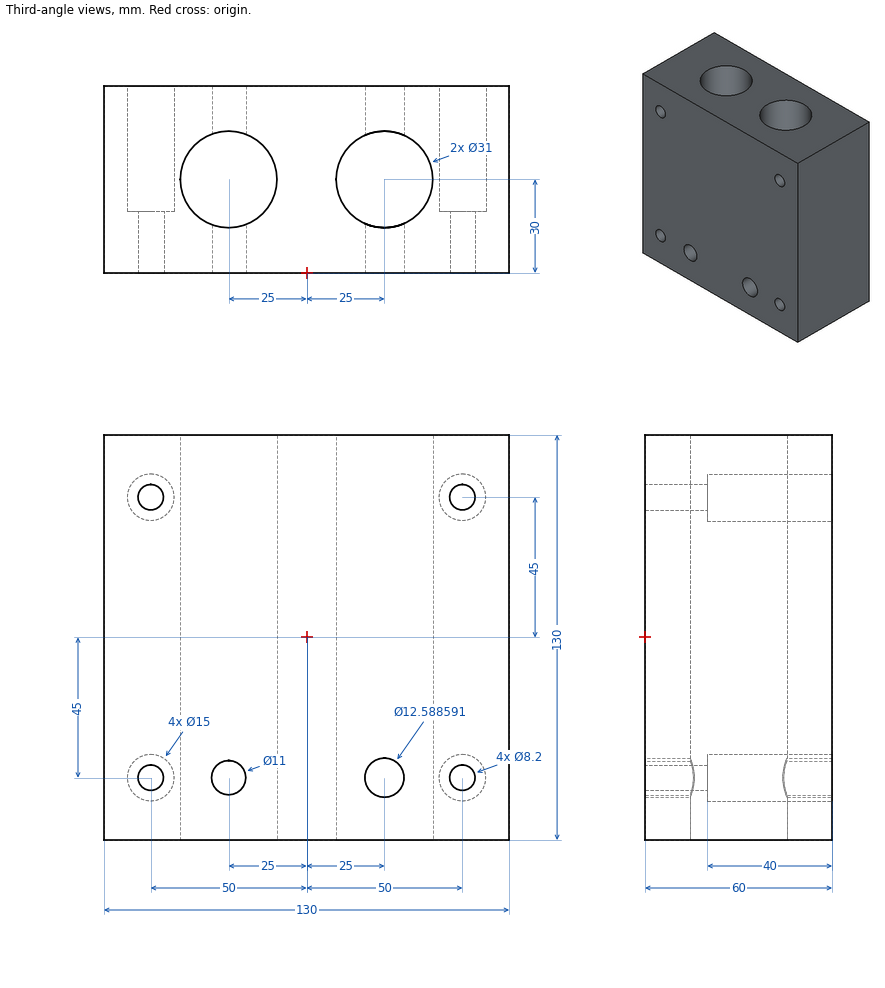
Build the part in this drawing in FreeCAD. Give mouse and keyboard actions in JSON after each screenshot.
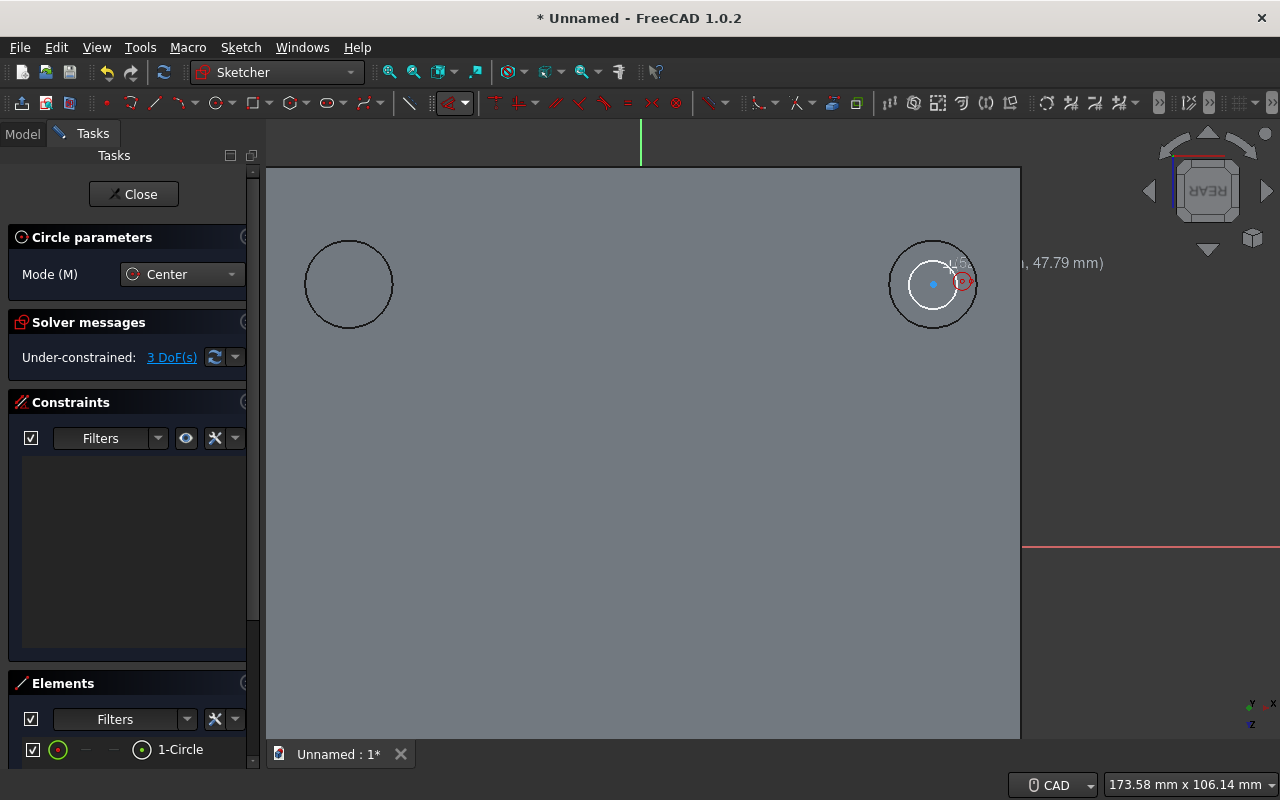
{"action": "left_click", "coordinate": [349, 284]}
{"action": "left_click", "coordinate": [366, 267]}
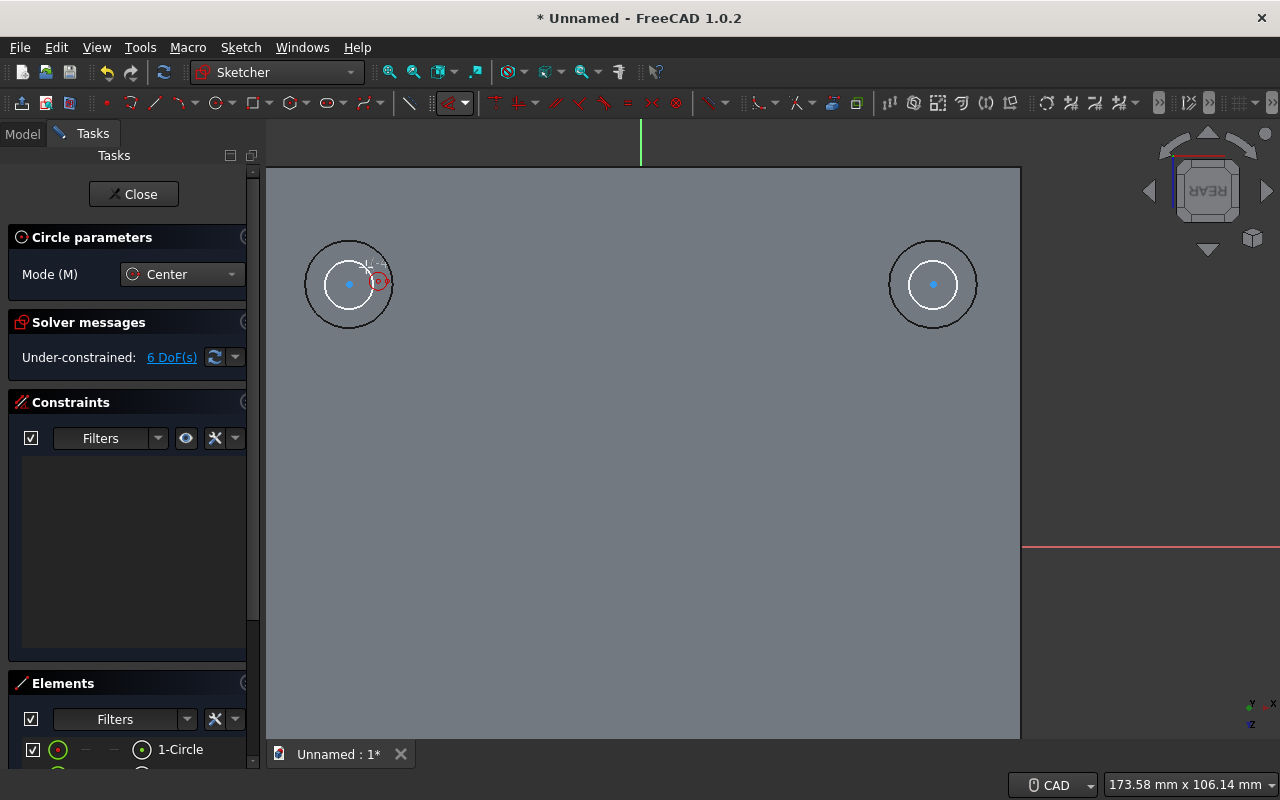
{"action": "scroll", "coordinate": [834, 189], "scroll_direction": "down", "scroll_amount": 2}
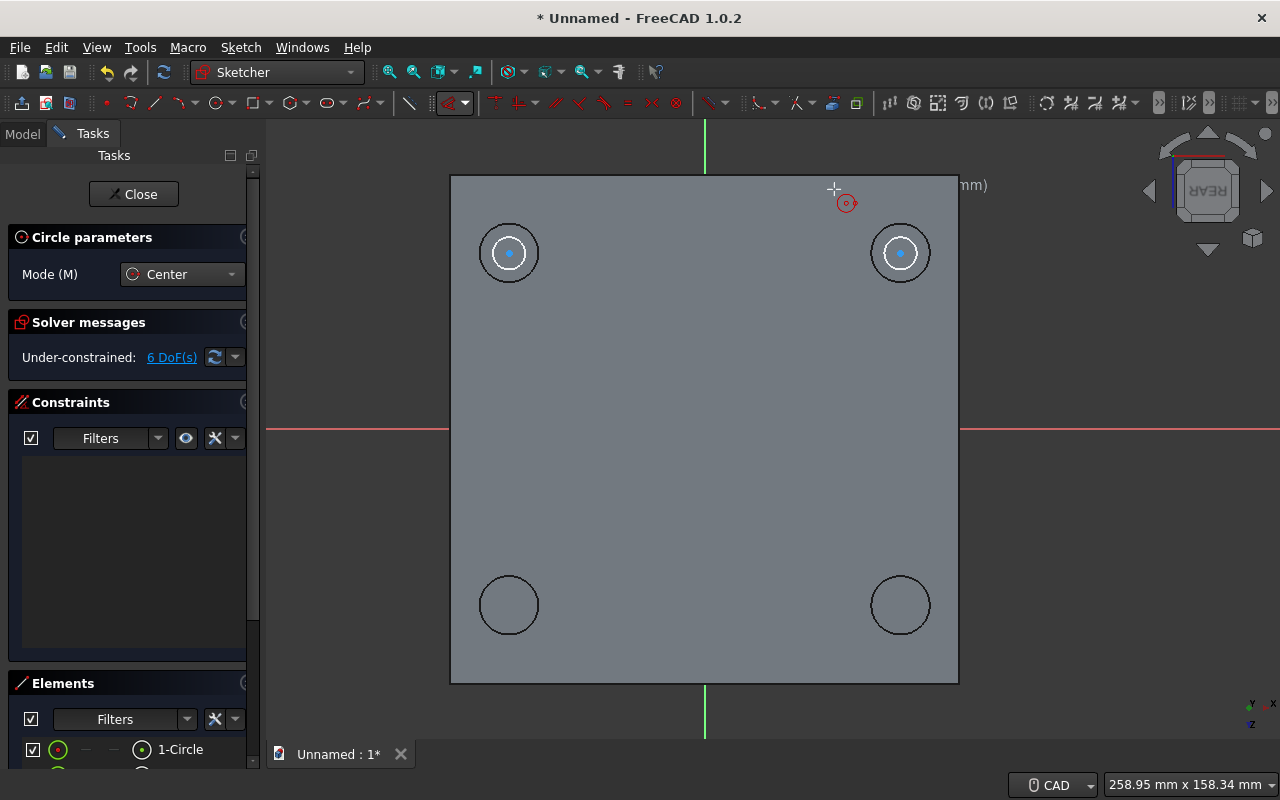
{"action": "scroll", "coordinate": [509, 605], "scroll_direction": "up", "scroll_amount": 2}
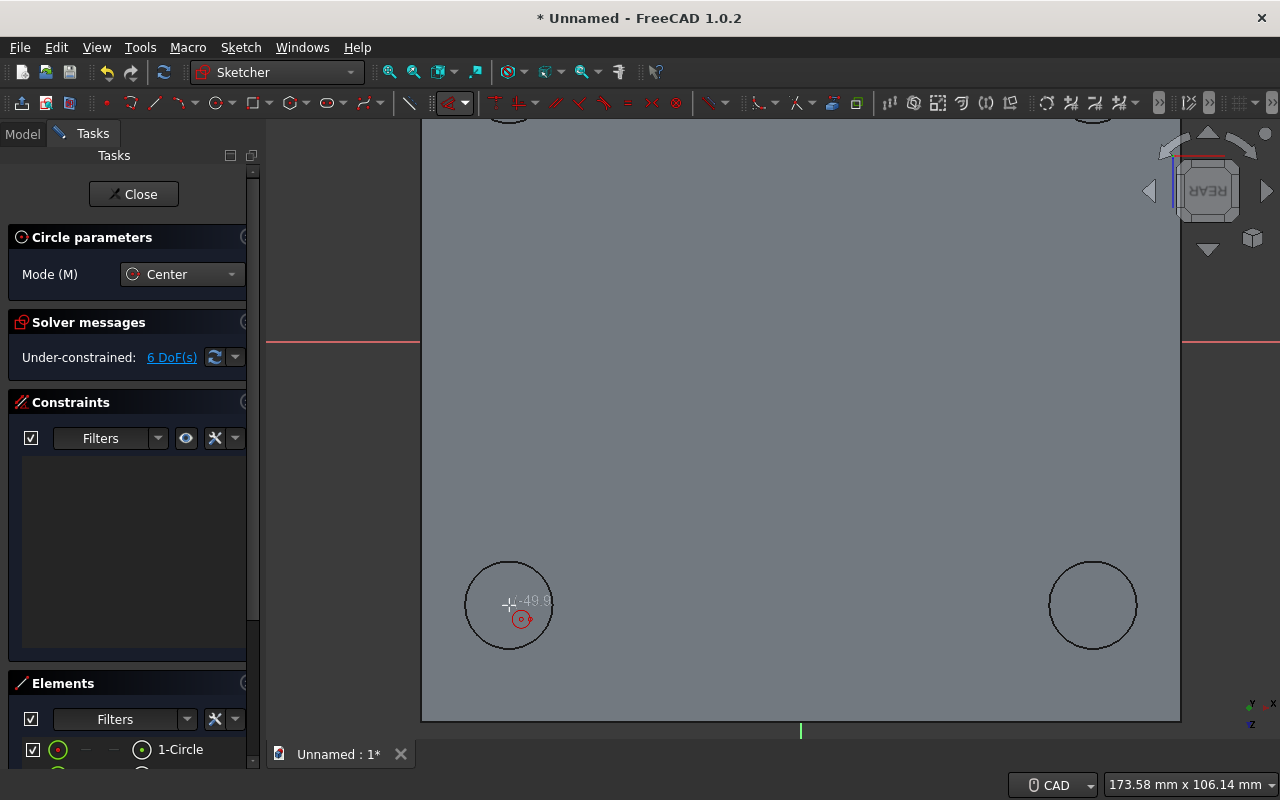
{"action": "left_click", "coordinate": [509, 605]}
{"action": "left_click", "coordinate": [526, 588]}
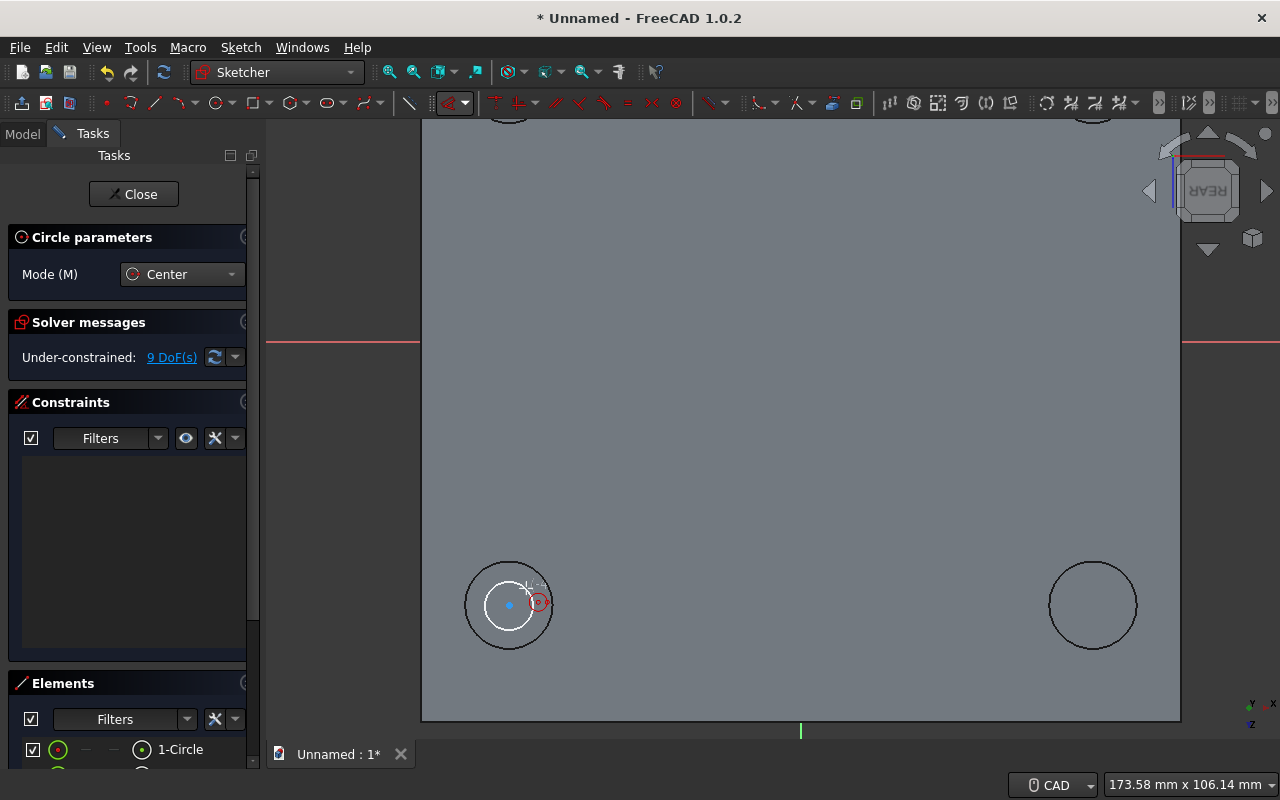
{"action": "left_click", "coordinate": [1093, 605]}
{"action": "left_click", "coordinate": [1110, 588]}
{"action": "key", "text": "Escape"}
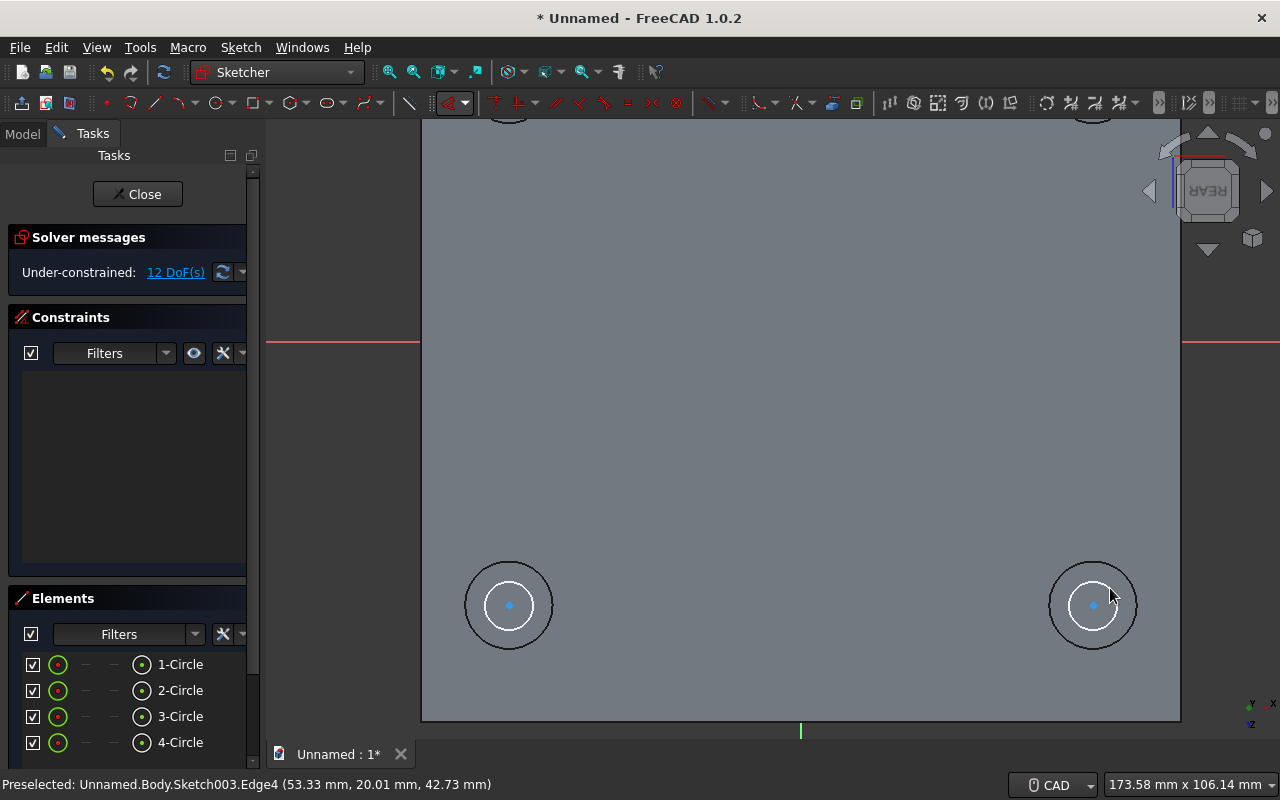
{"action": "scroll", "coordinate": [508, 605], "scroll_direction": "down", "scroll_amount": 2}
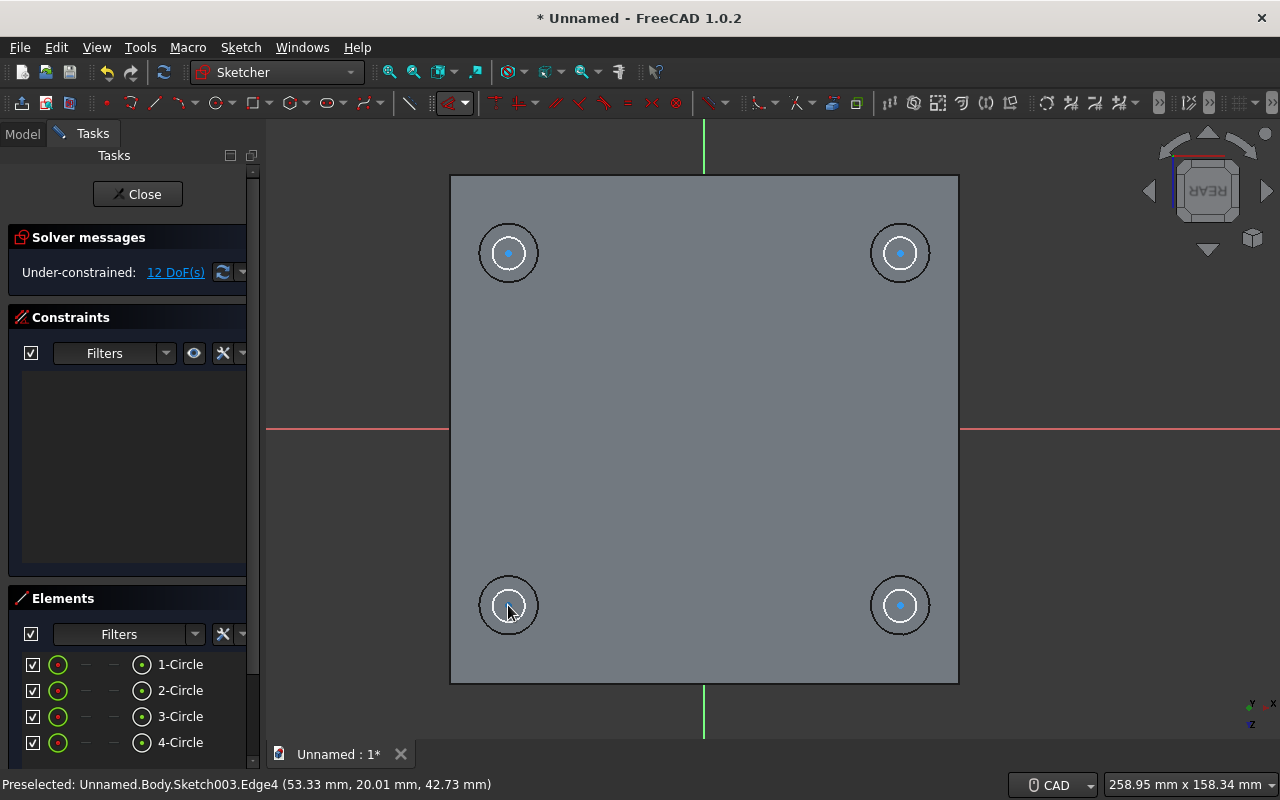
{"action": "left_click", "coordinate": [912, 242]}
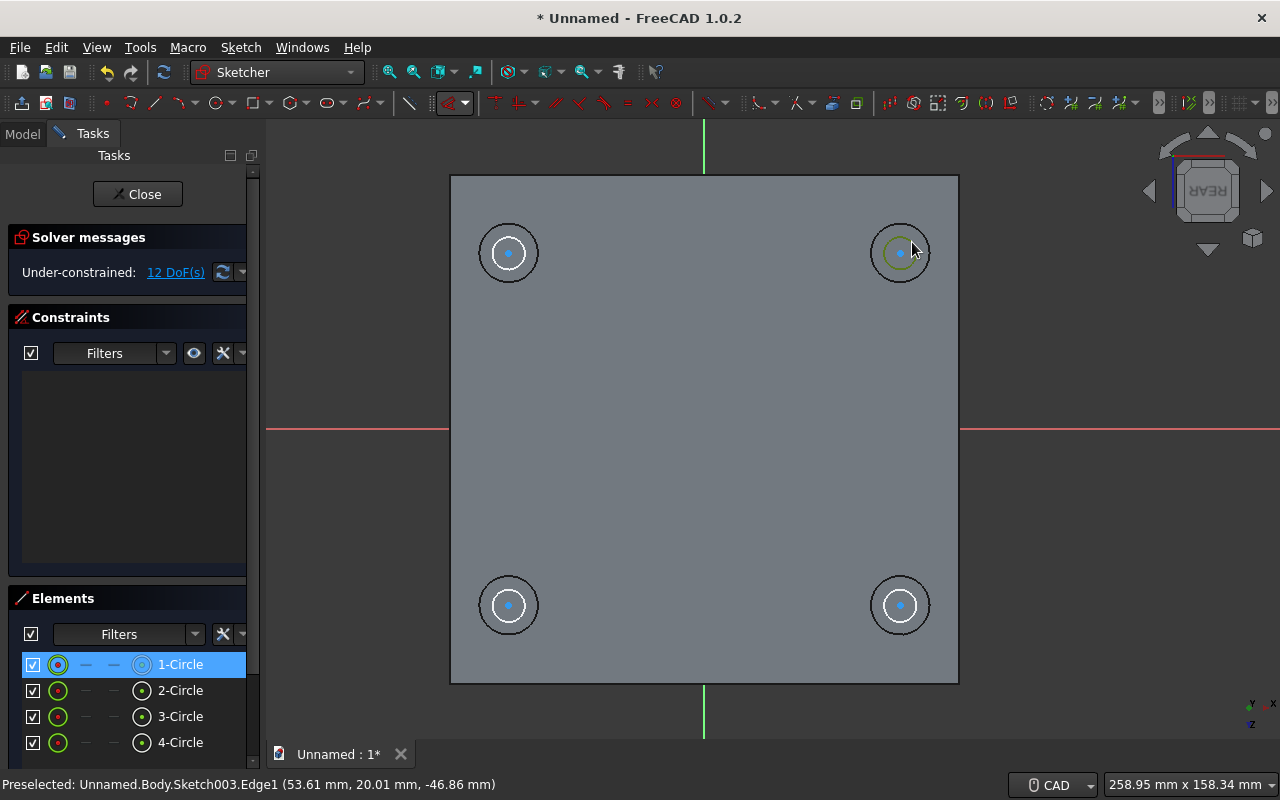
{"action": "left_click", "coordinate": [520, 242]}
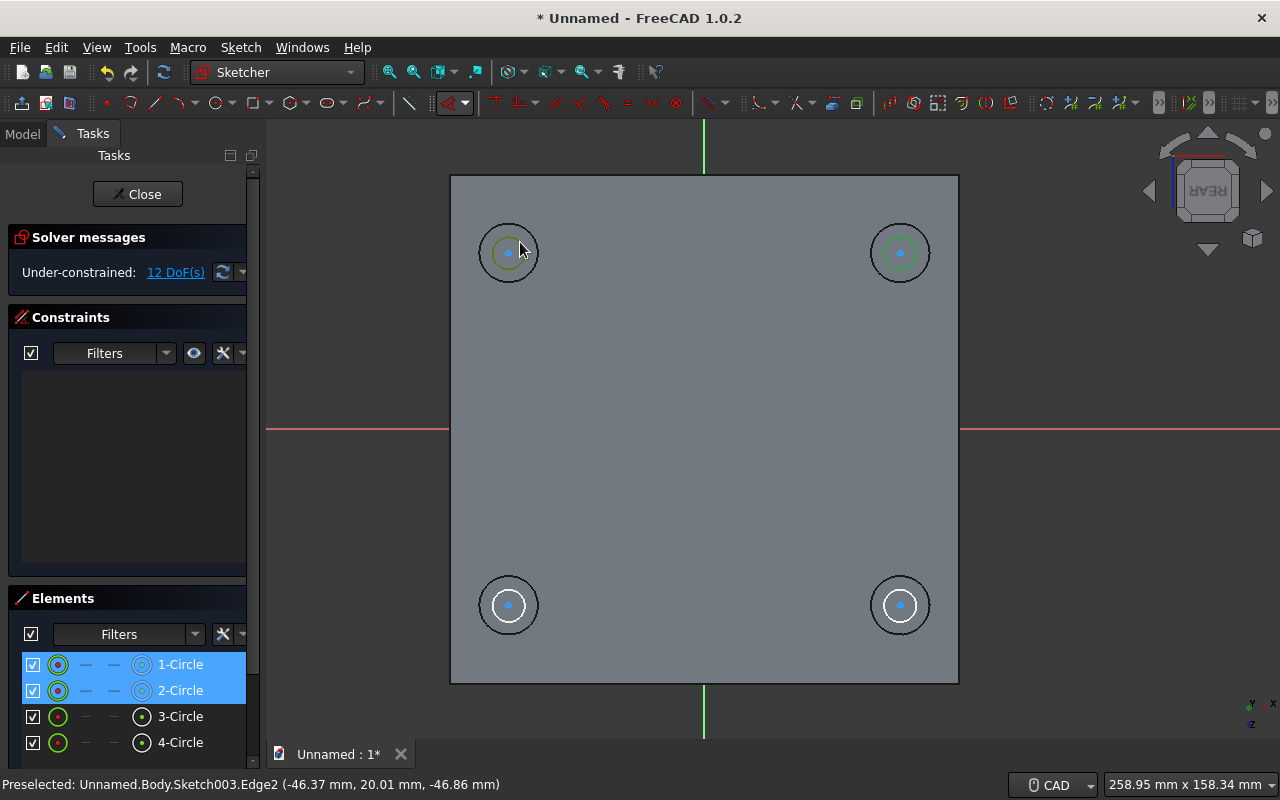
{"action": "left_click", "coordinate": [520, 594]}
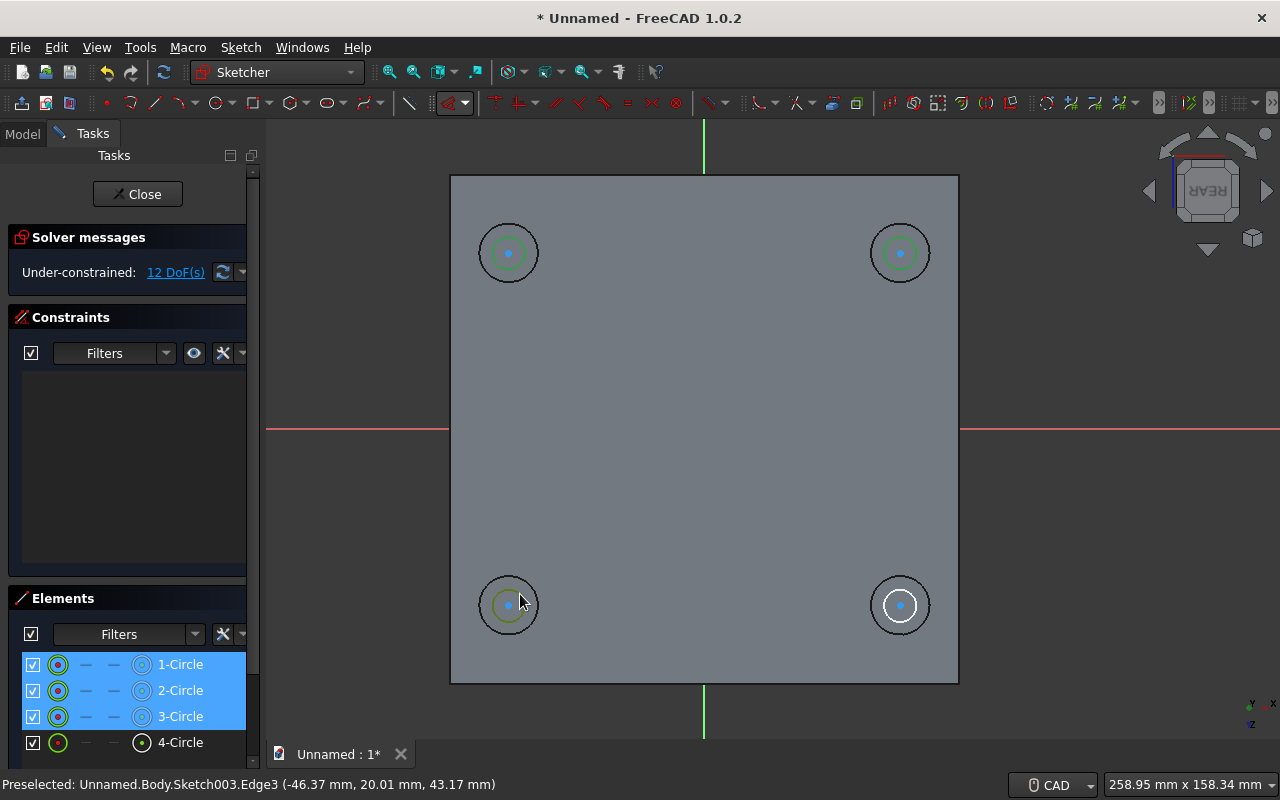
{"action": "left_click", "coordinate": [912, 594]}